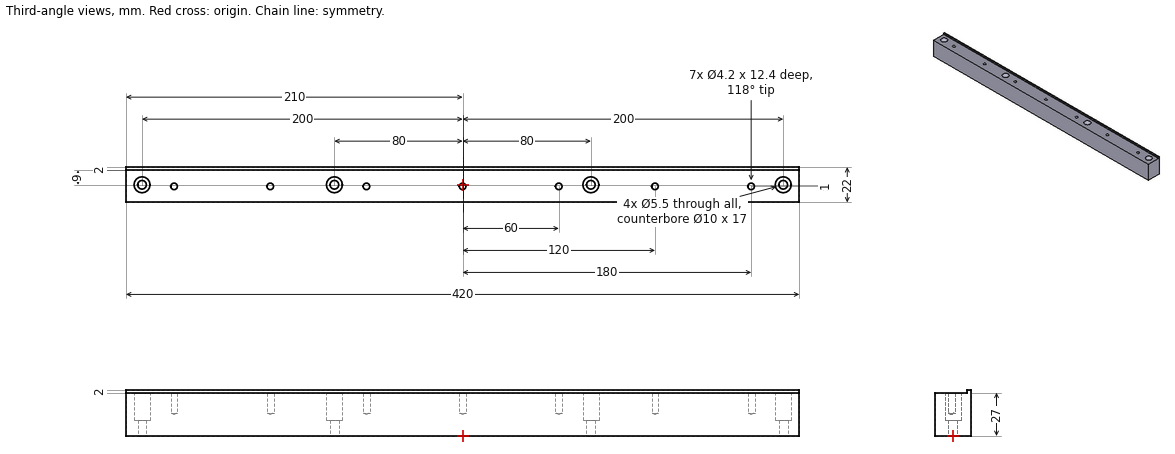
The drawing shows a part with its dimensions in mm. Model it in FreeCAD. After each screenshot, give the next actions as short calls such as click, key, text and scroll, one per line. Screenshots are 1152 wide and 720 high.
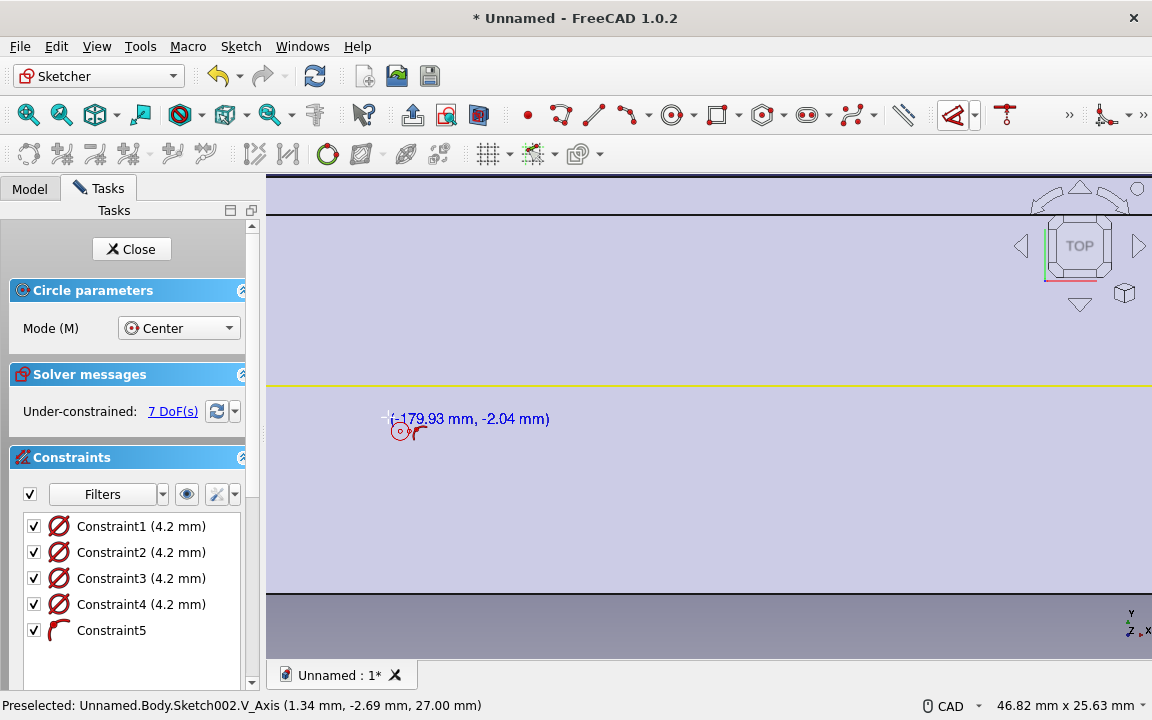
click(385, 405)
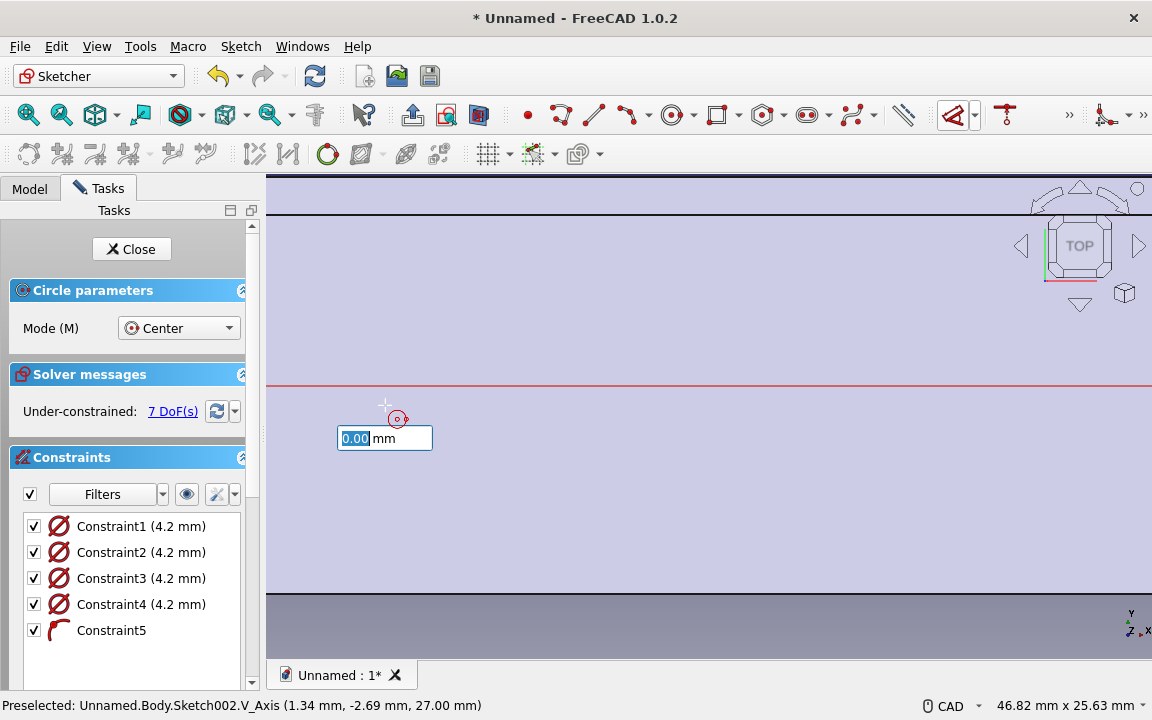
scroll(388, 417, down, 13)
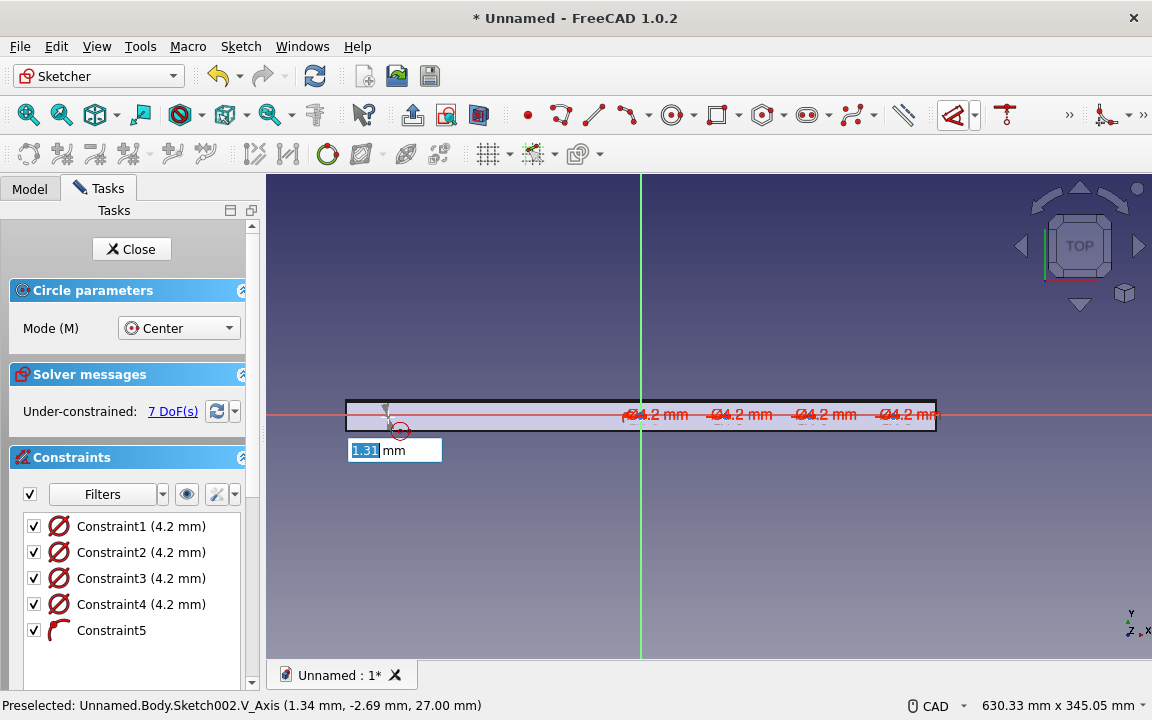
scroll(390, 419, up, 8)
move(389, 415)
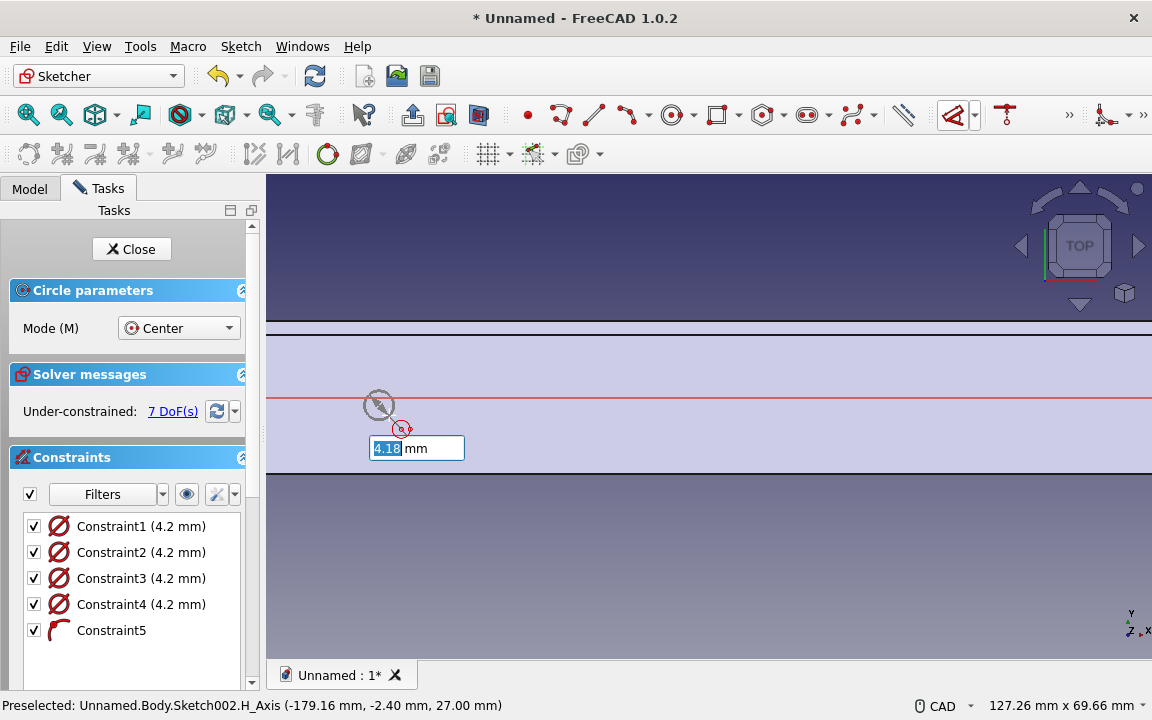
text(4.2)
key(Return)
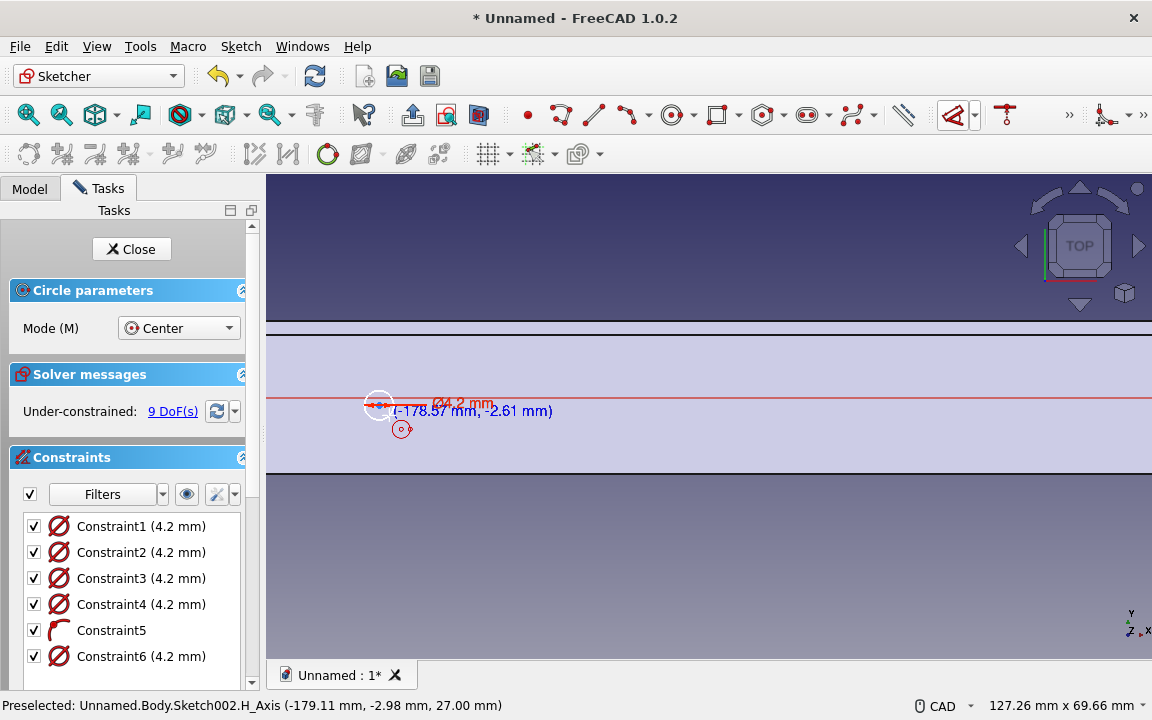
scroll(797, 405, up, 5)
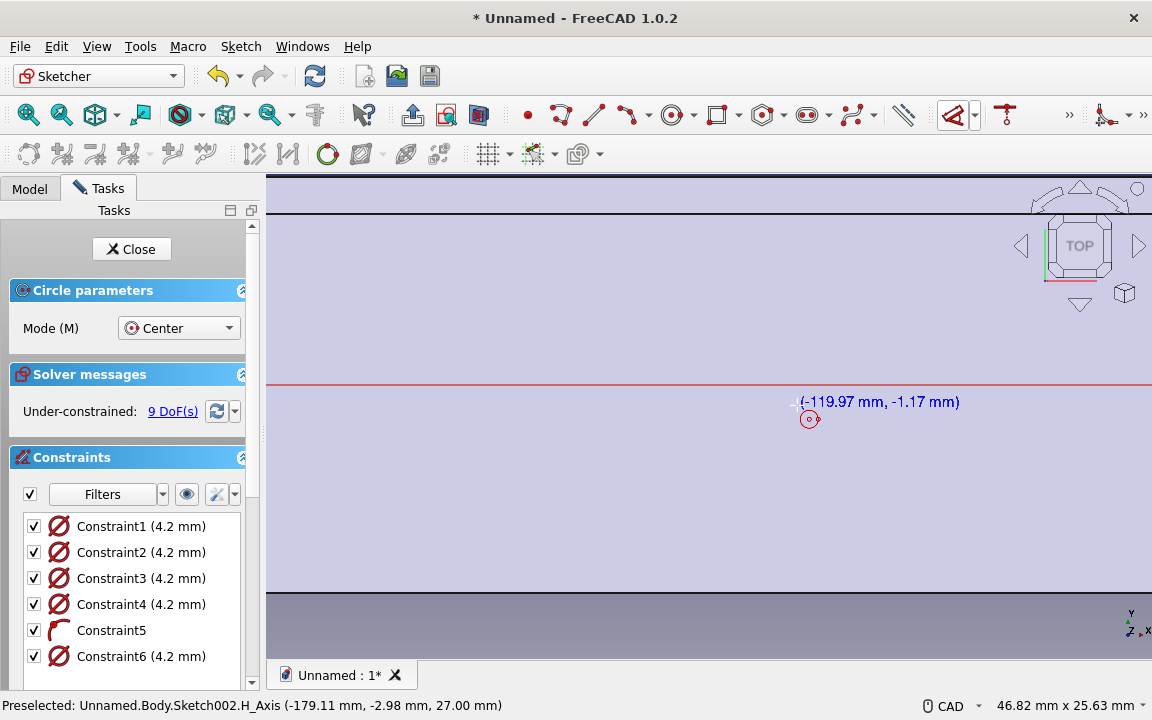
click(795, 404)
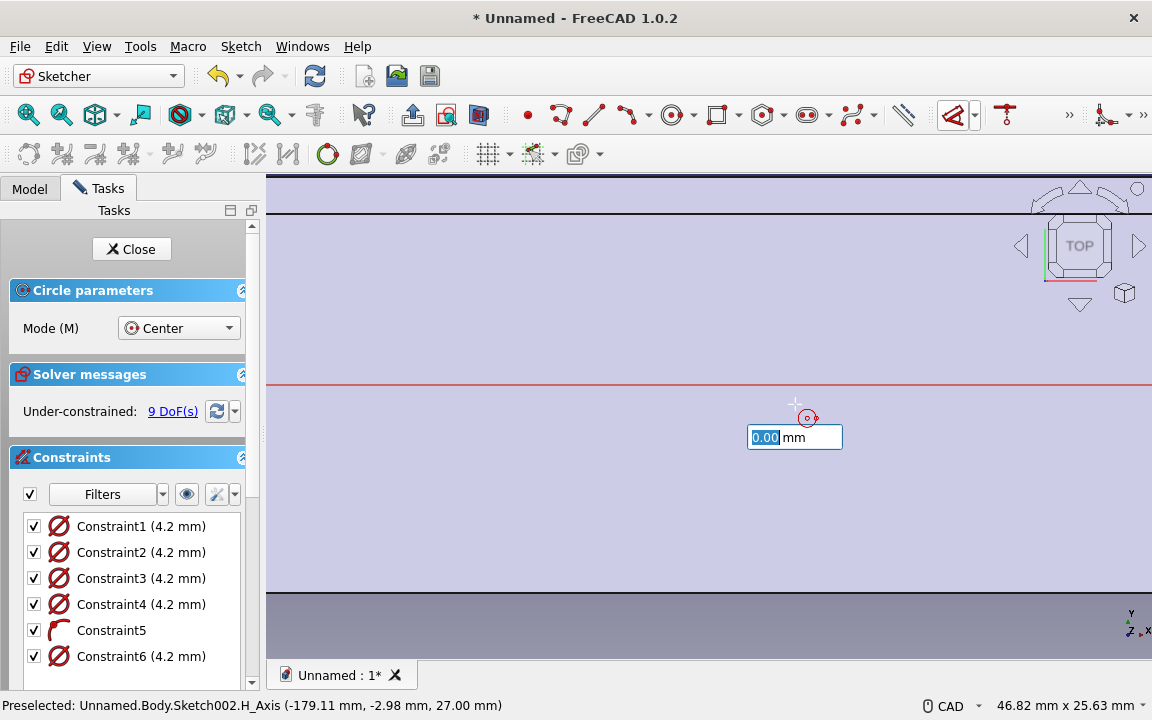
scroll(446, 418, down, 13)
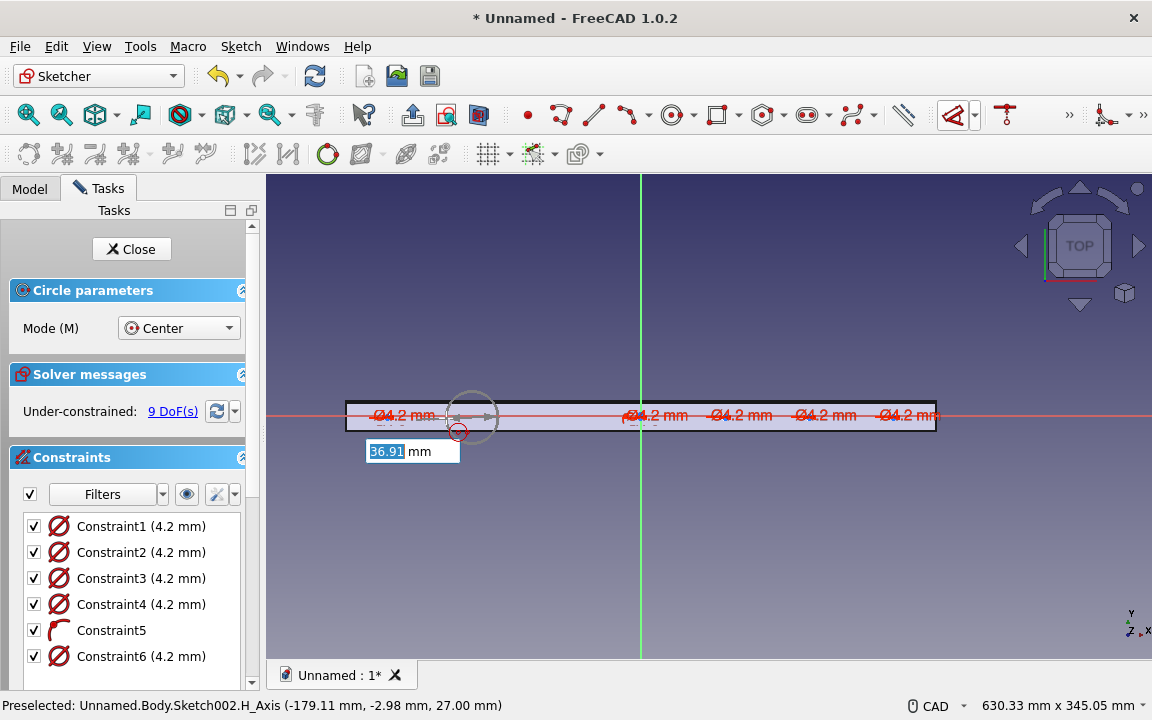
scroll(474, 419, up, 8)
move(474, 419)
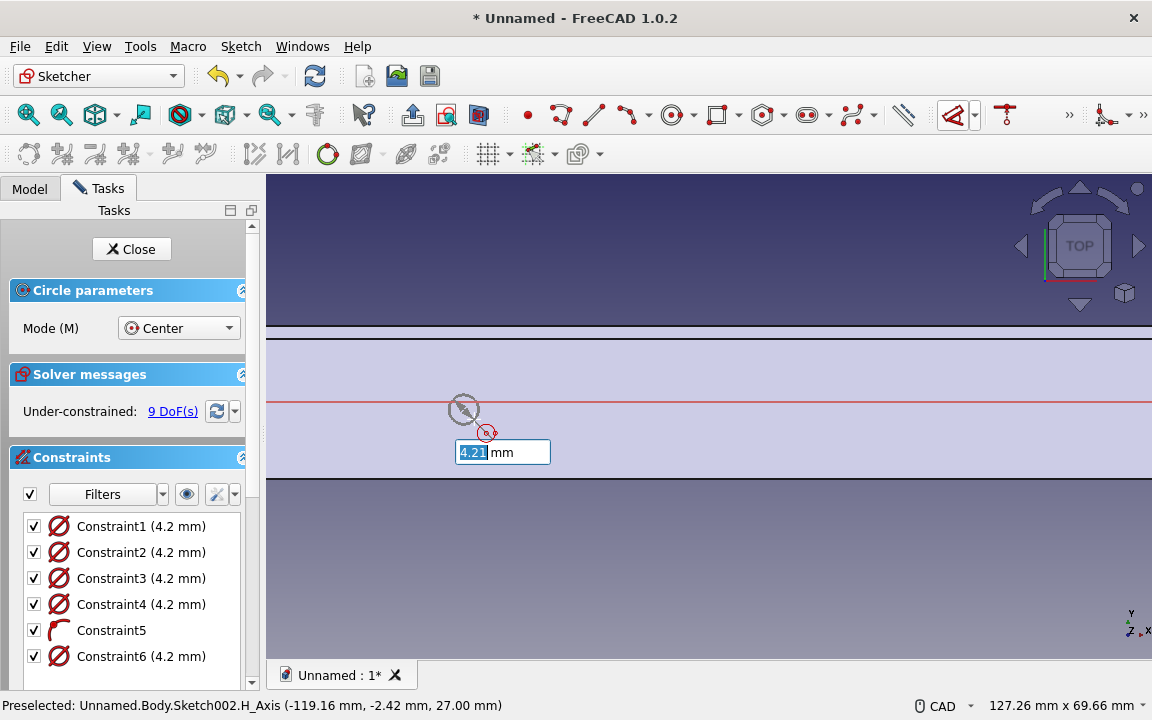
text(4.2)
key(Return)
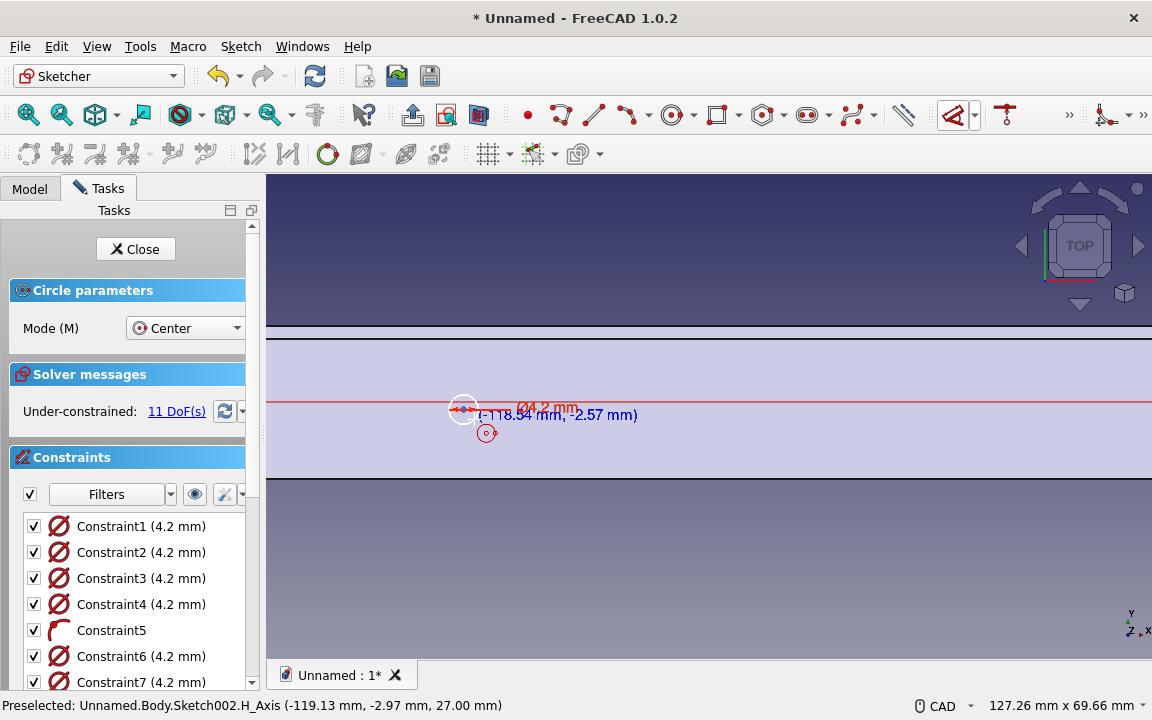
scroll(882, 409, up, 5)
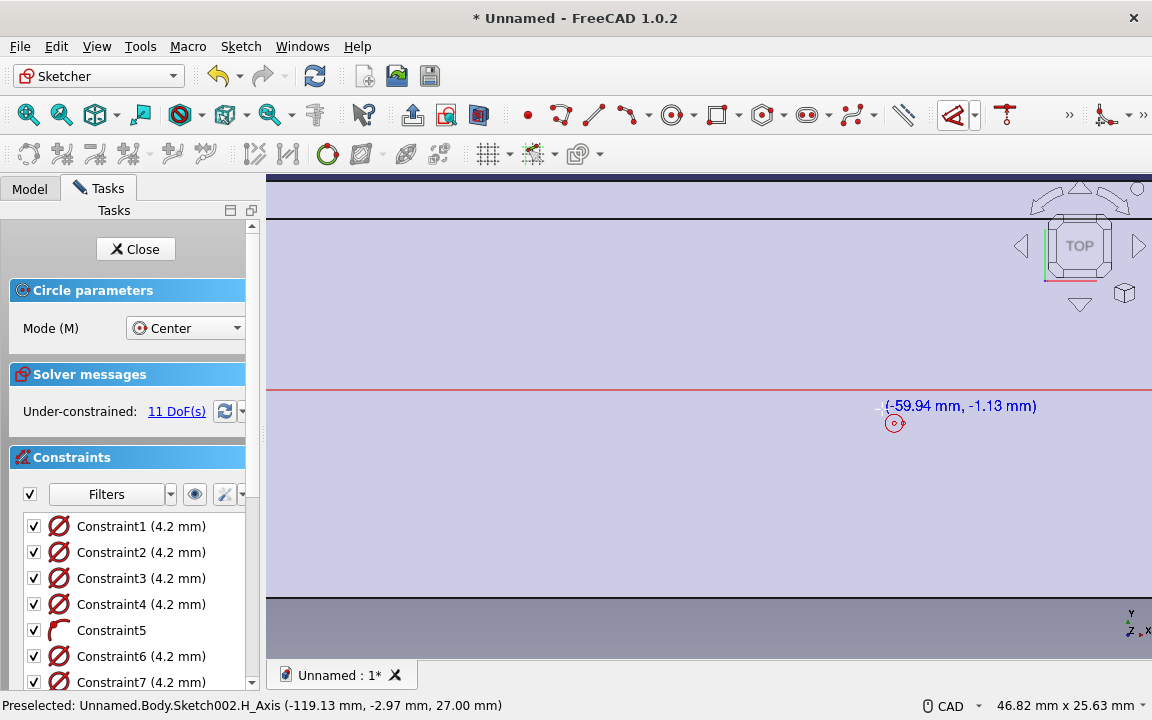
click(880, 408)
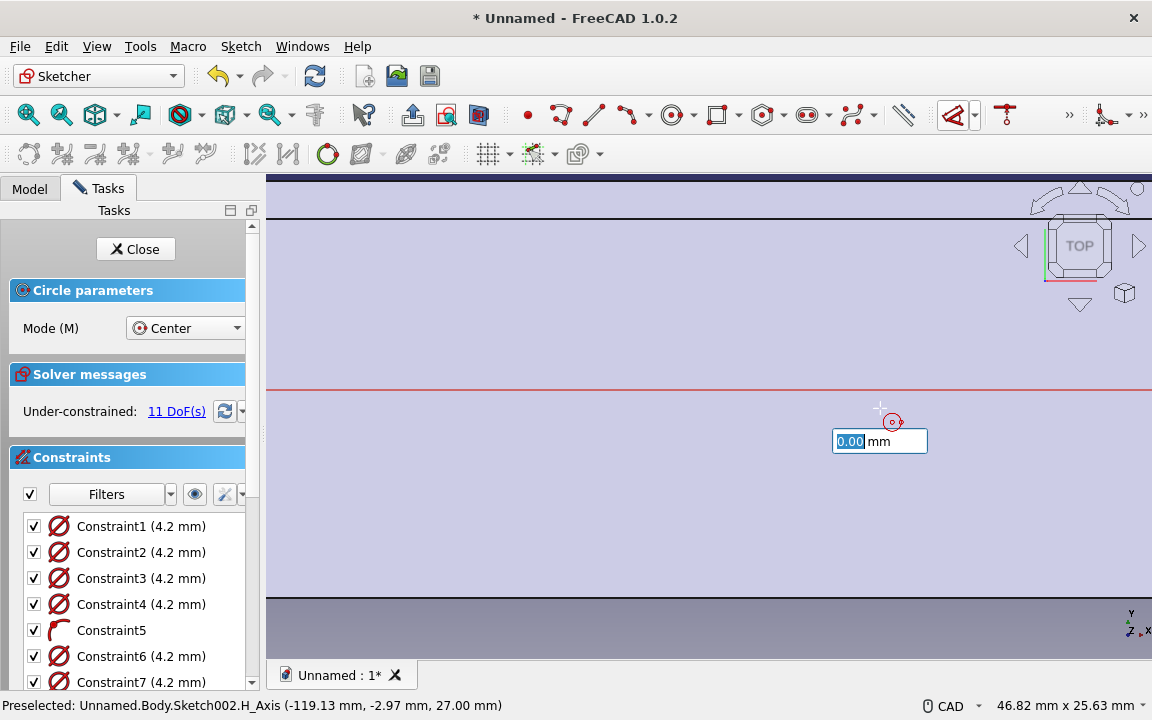
scroll(530, 417, down, 13)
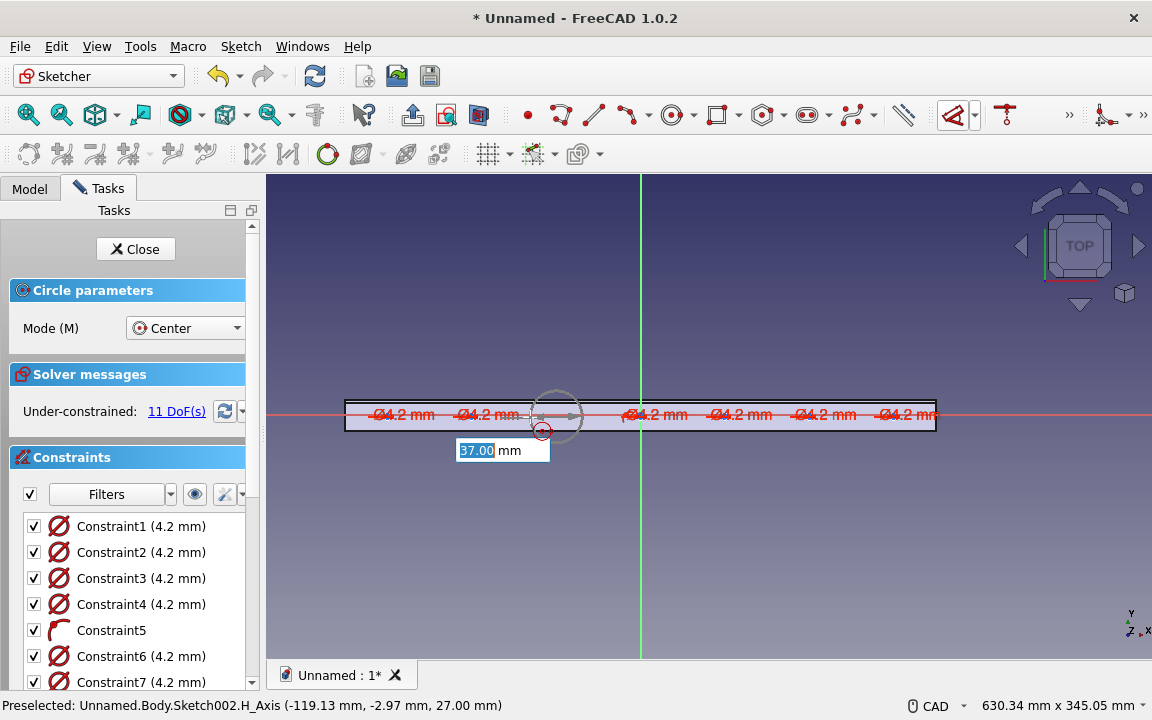
scroll(558, 419, up, 8)
move(558, 417)